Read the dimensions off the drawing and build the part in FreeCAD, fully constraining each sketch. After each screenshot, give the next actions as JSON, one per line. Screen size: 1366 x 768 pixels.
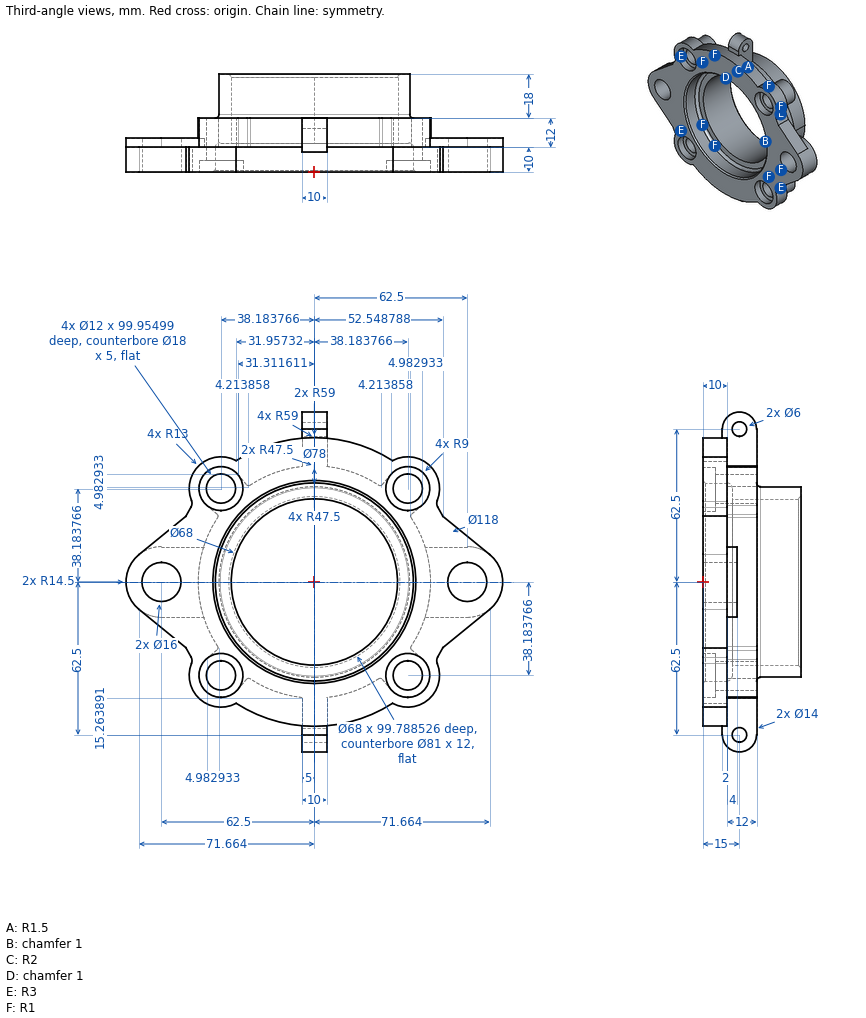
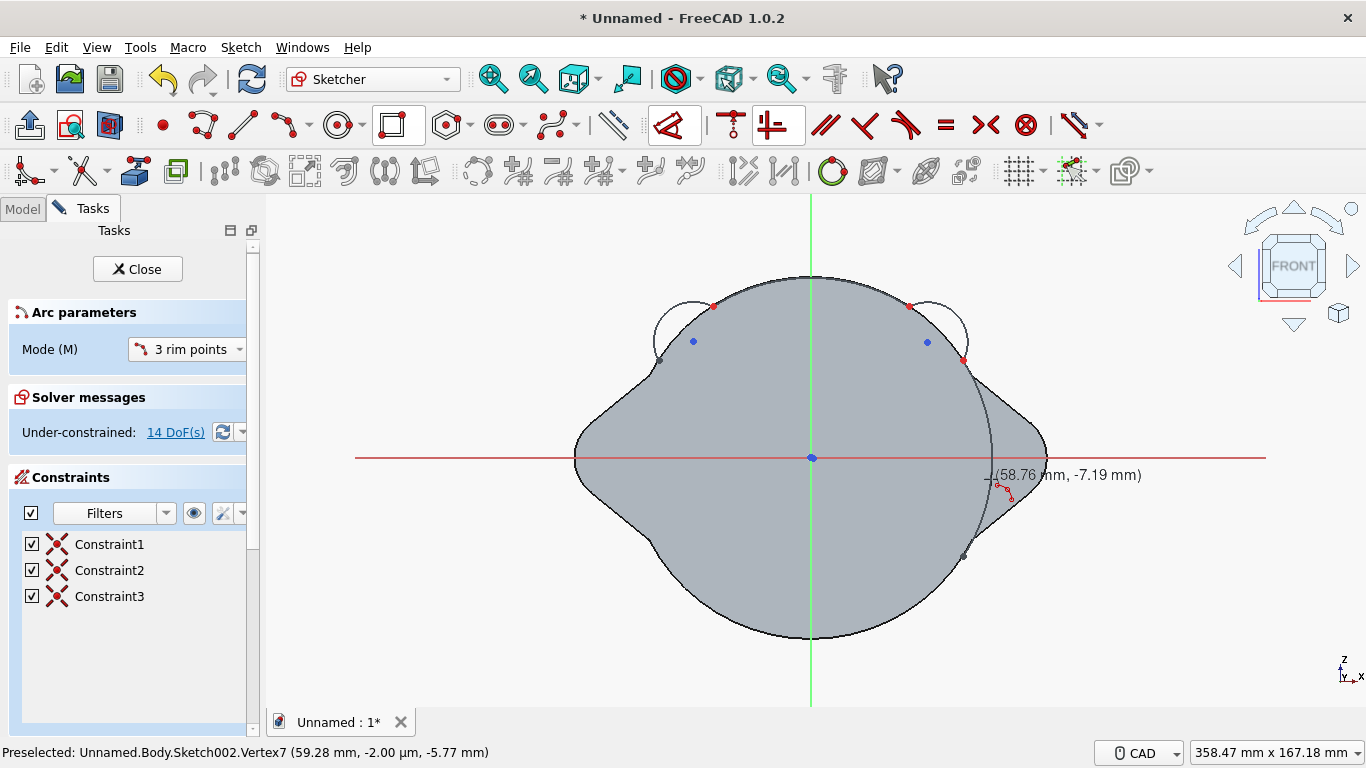
{"action": "left_click", "coordinate": [963, 557]}
{"action": "left_click", "coordinate": [909, 610]}
{"action": "left_click", "coordinate": [956, 603]}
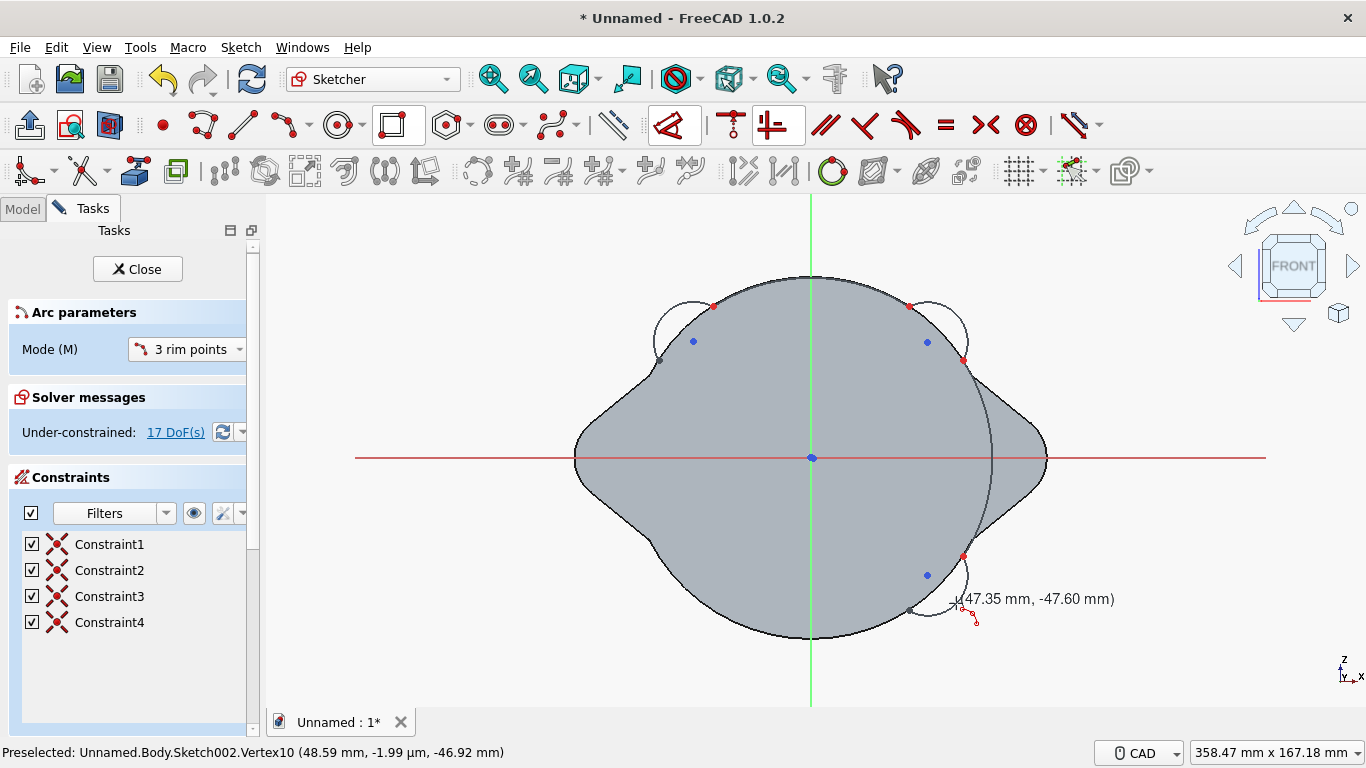
{"action": "left_click", "coordinate": [909, 611]}
{"action": "left_click", "coordinate": [713, 610]}
{"action": "left_click", "coordinate": [790, 638]}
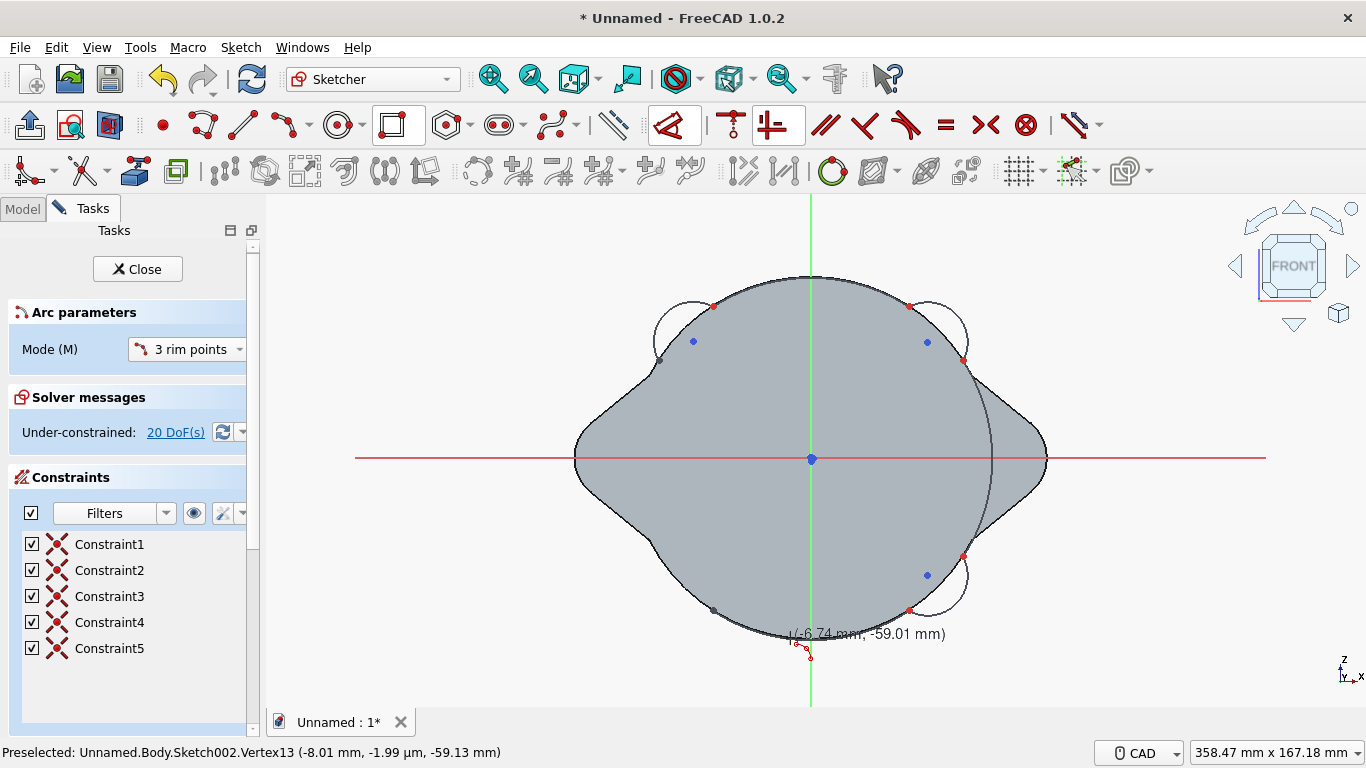
{"action": "left_click", "coordinate": [713, 611]}
{"action": "left_click", "coordinate": [659, 556]}
{"action": "left_click", "coordinate": [665, 603]}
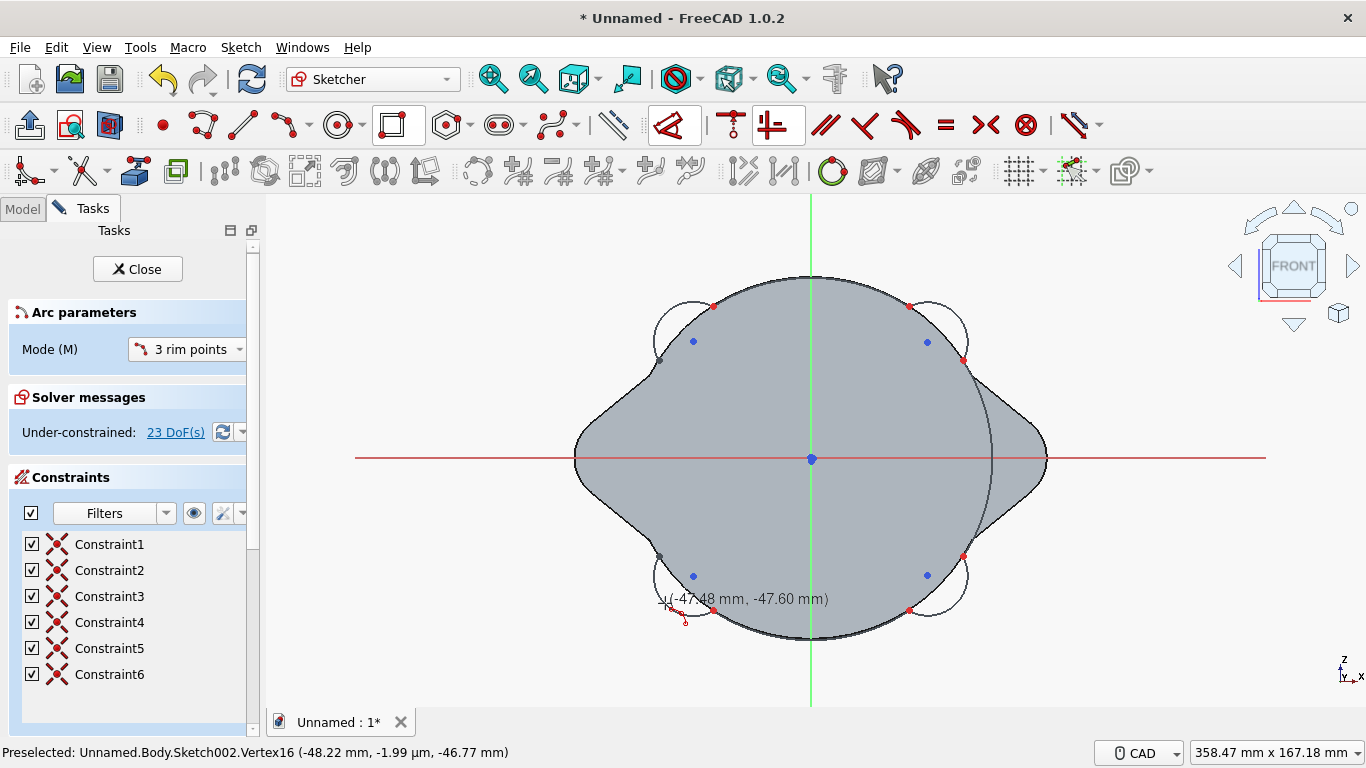
{"action": "left_click", "coordinate": [659, 557]}
{"action": "left_click", "coordinate": [659, 361]}
{"action": "left_click", "coordinate": [631, 437]}
{"action": "key", "text": "Escape"}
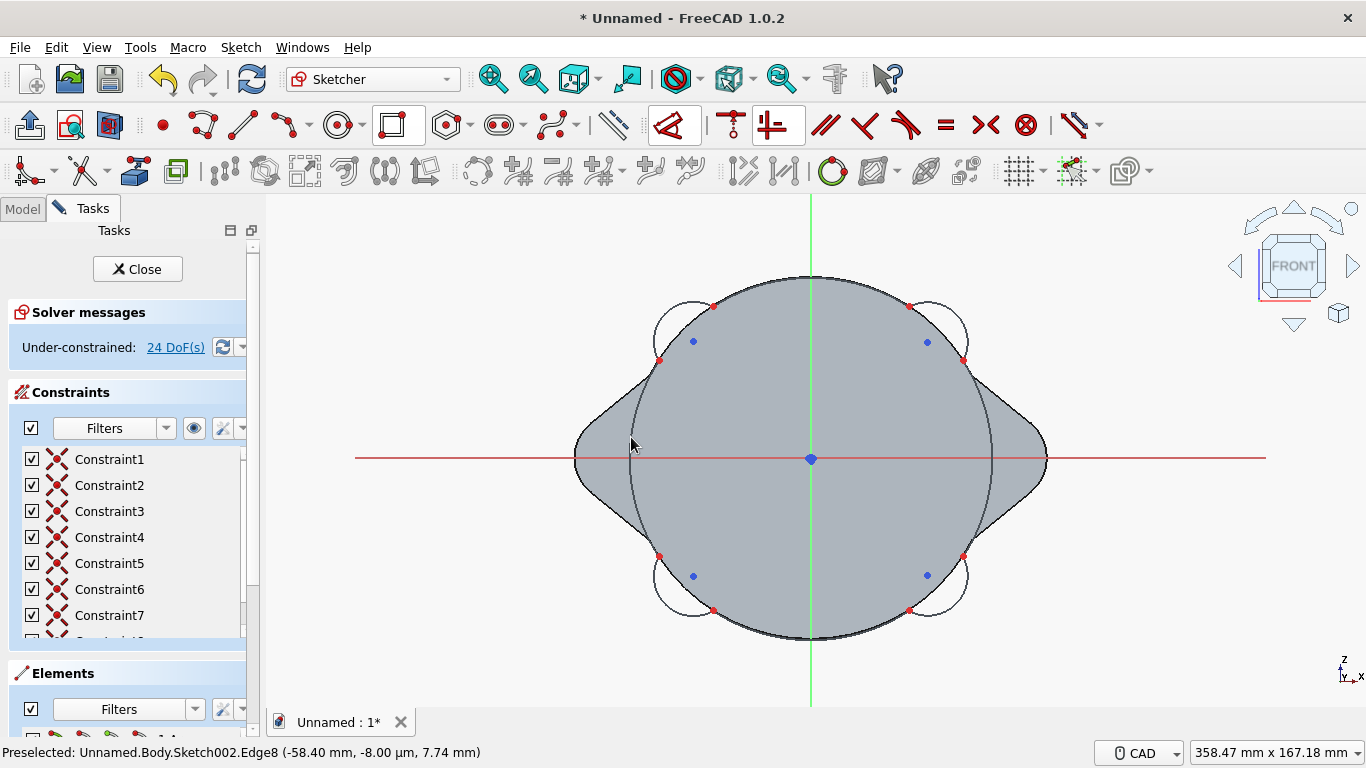
{"action": "left_click", "coordinate": [852, 283]}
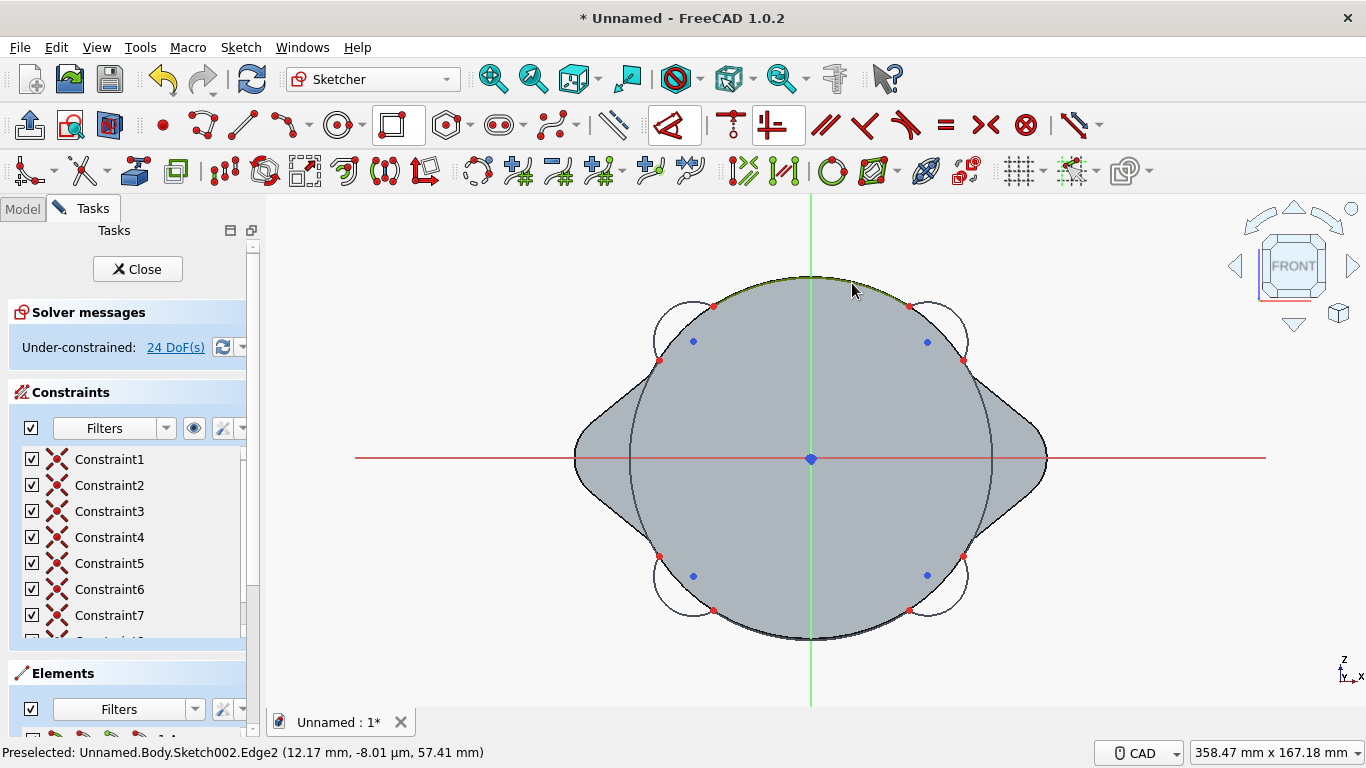
{"action": "left_click", "coordinate": [987, 500]}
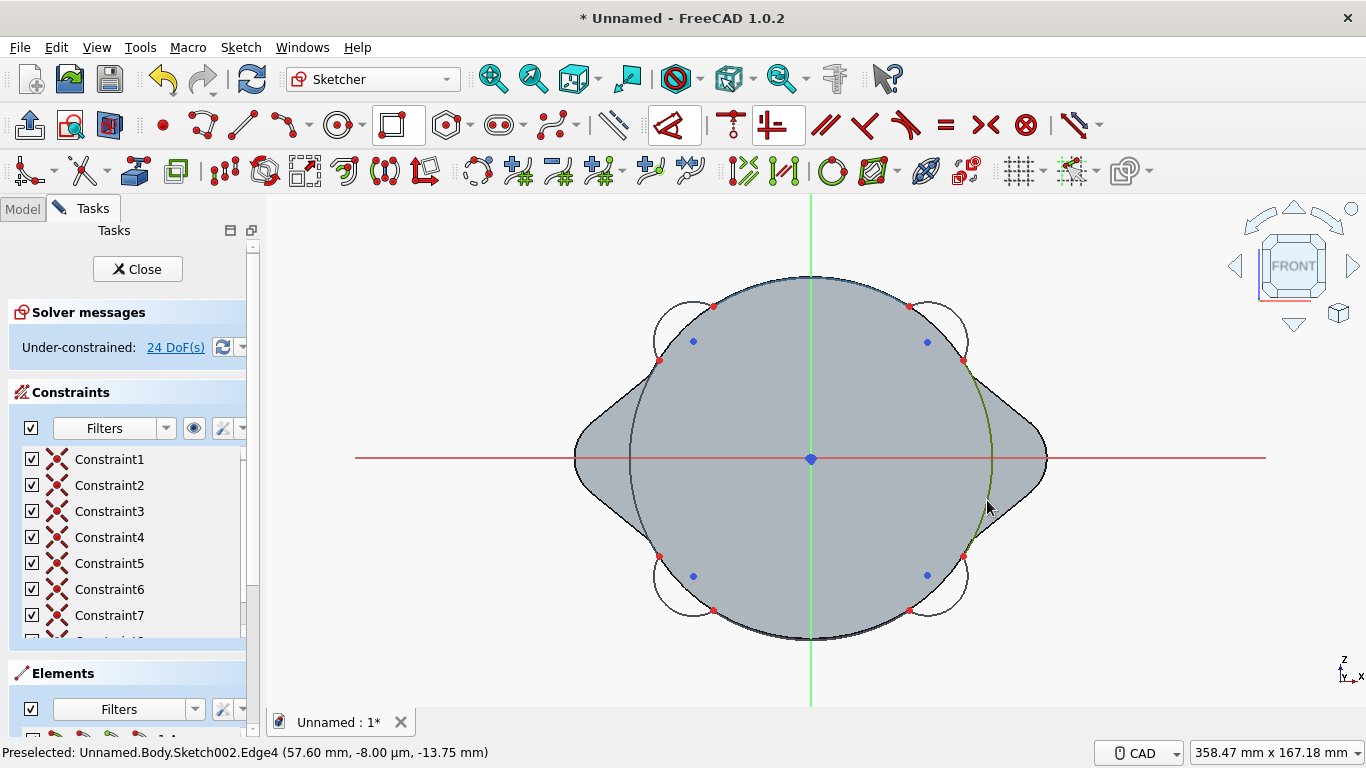
{"action": "left_click", "coordinate": [732, 126]}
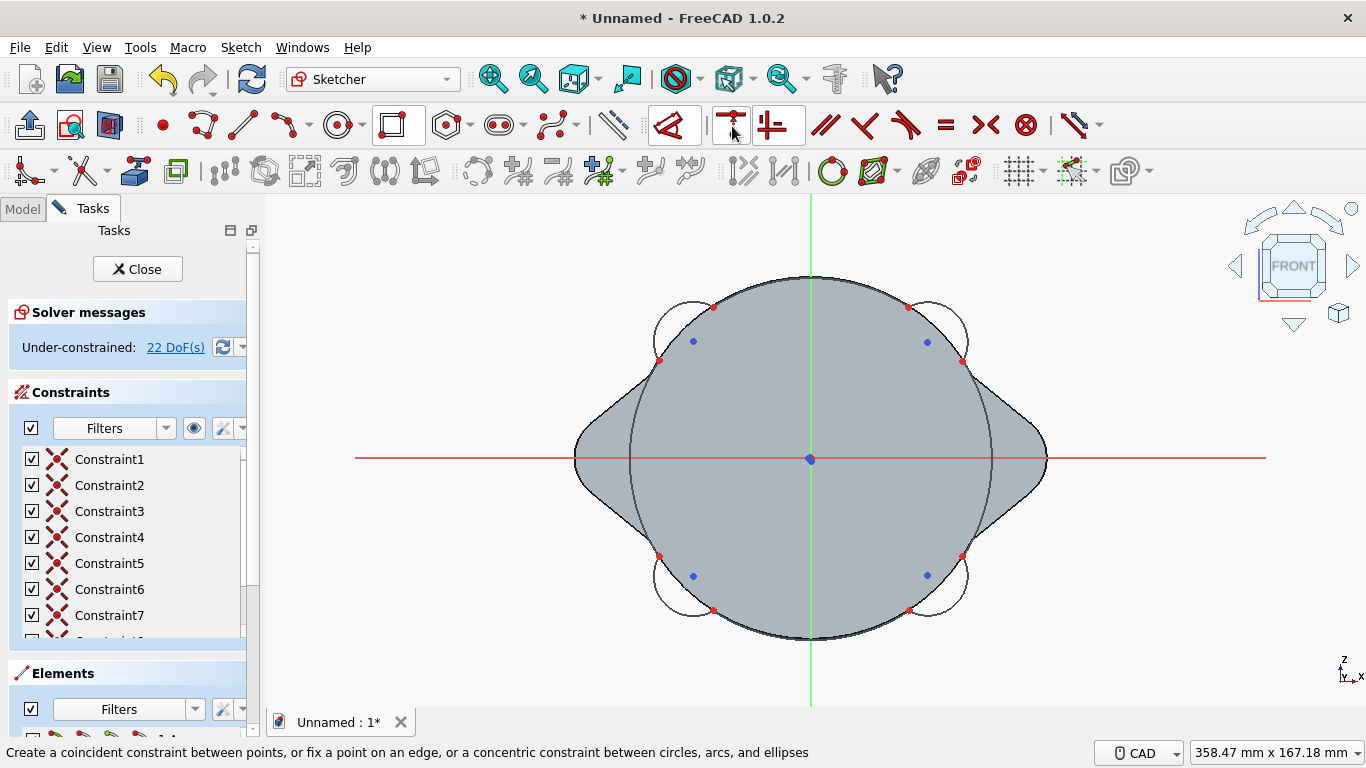
{"action": "left_click", "coordinate": [852, 283]}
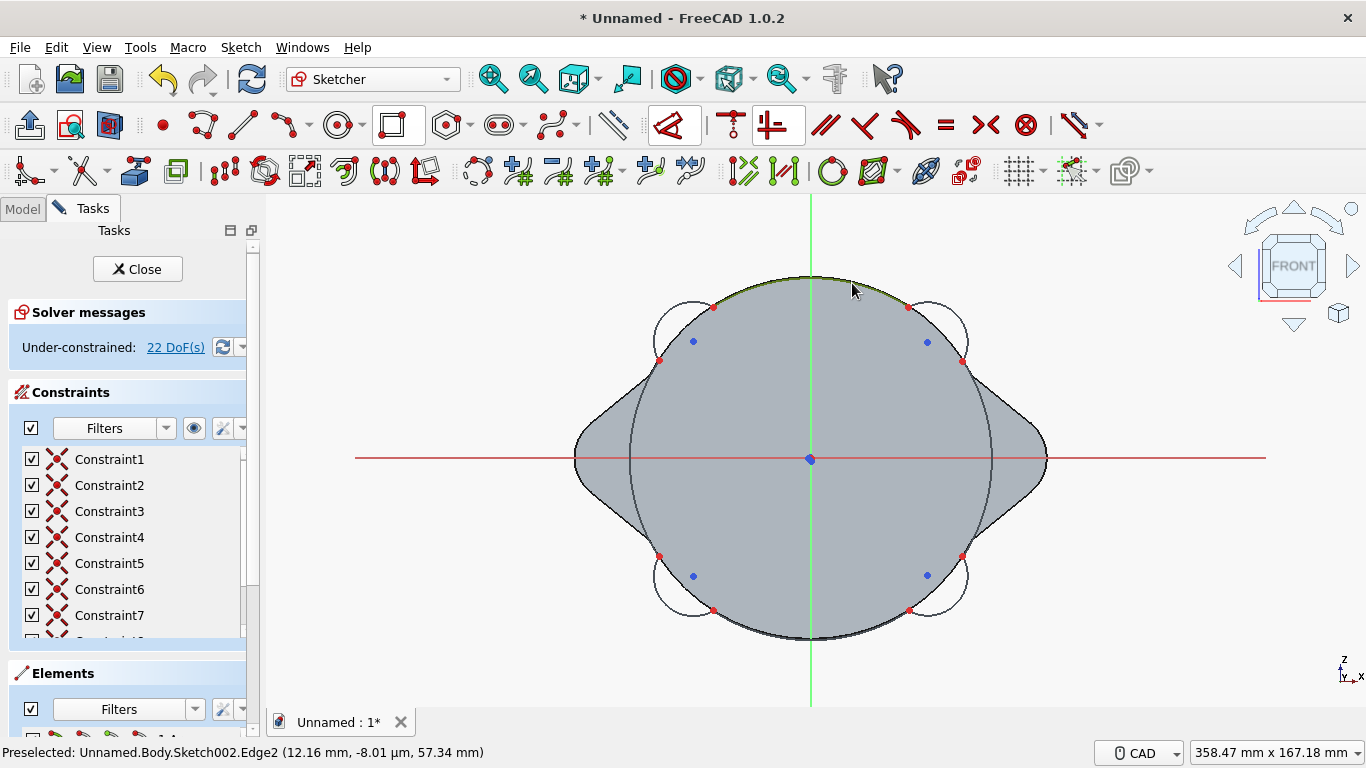
{"action": "left_click", "coordinate": [770, 635]}